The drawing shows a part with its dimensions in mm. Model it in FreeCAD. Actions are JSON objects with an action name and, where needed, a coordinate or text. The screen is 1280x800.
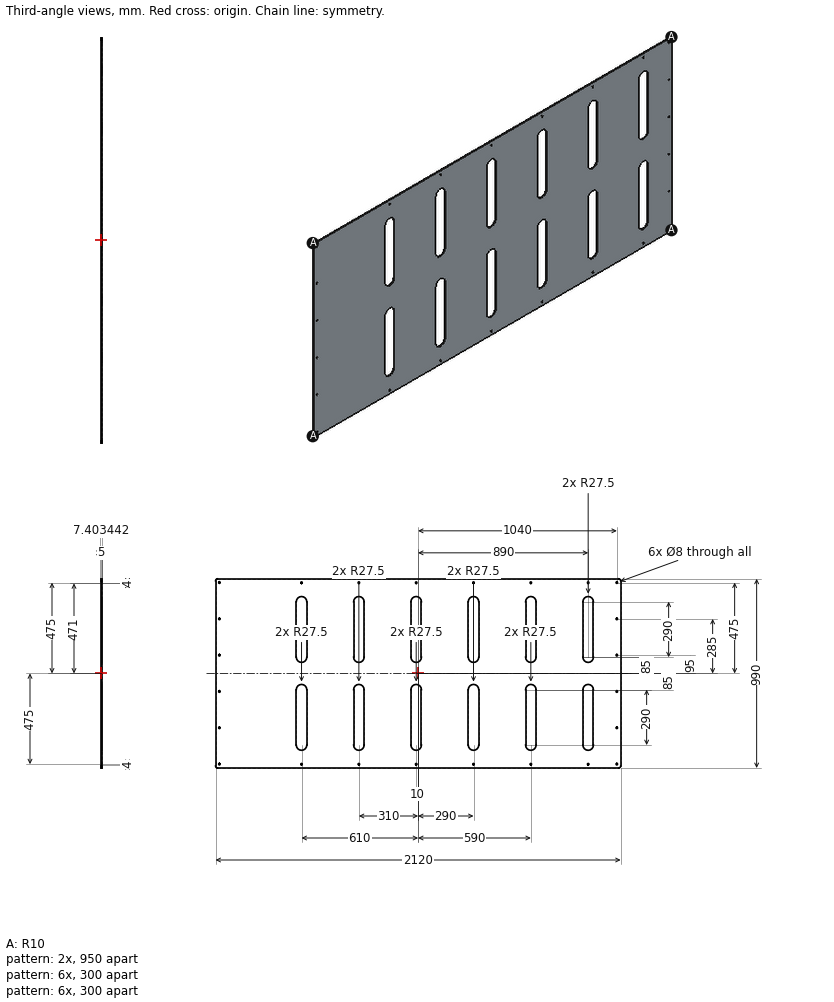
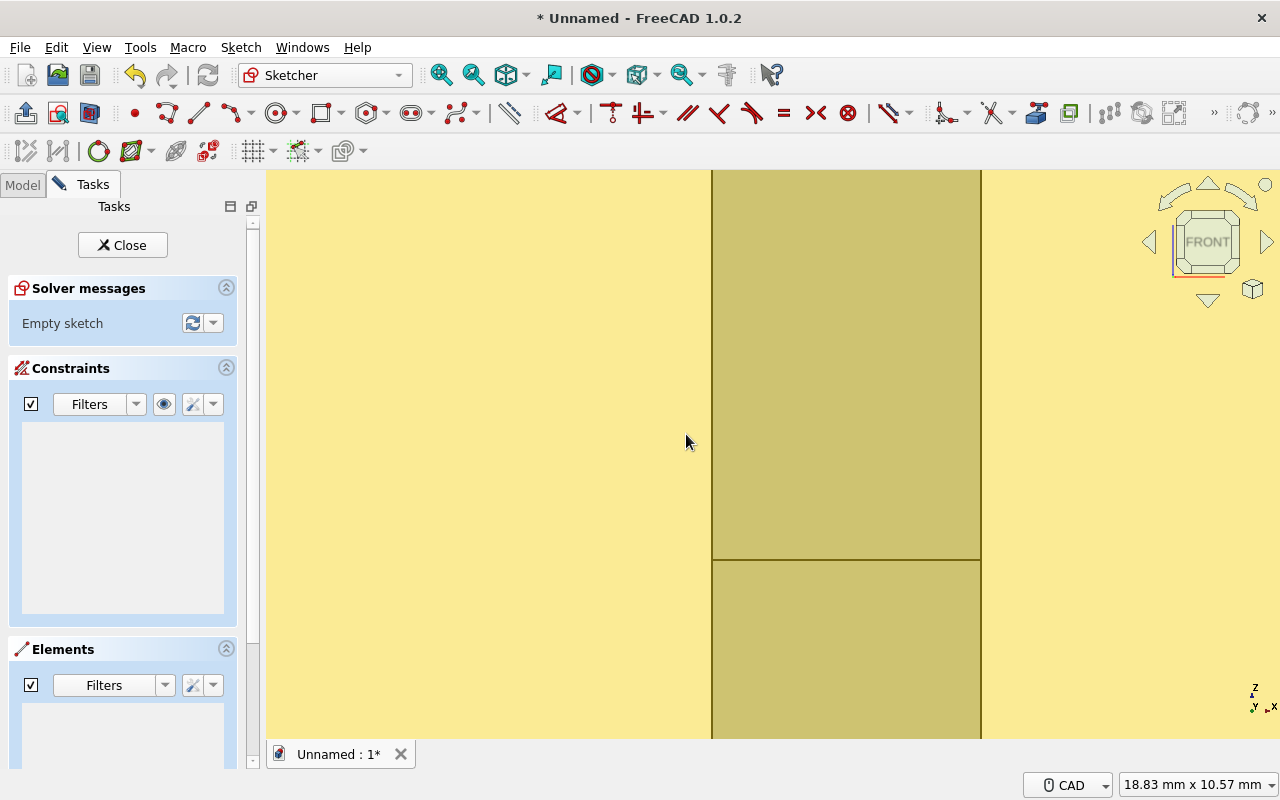
{"action": "left_click", "coordinate": [168, 114]}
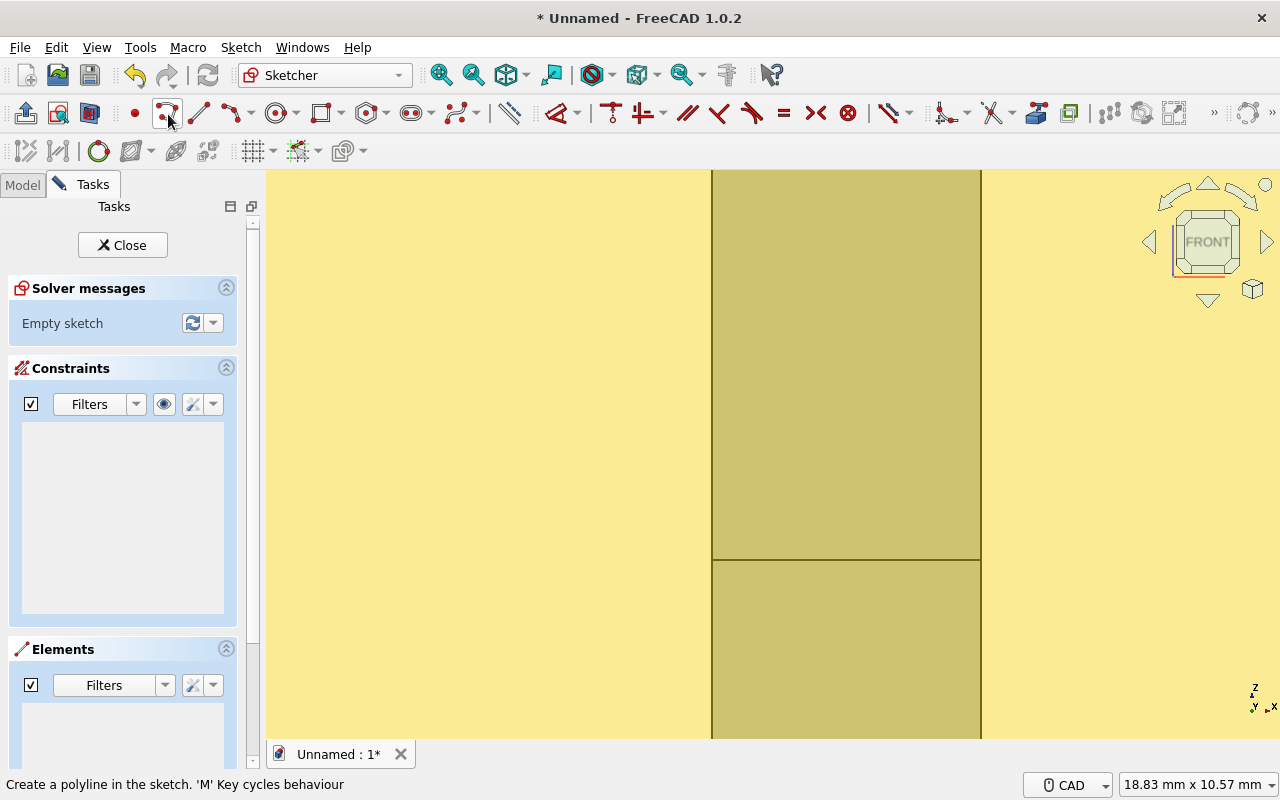
{"action": "left_click", "coordinate": [582, 345]}
{"action": "left_click", "coordinate": [981, 345]}
{"action": "left_click", "coordinate": [981, 560]}
{"action": "left_click", "coordinate": [712, 560]}
{"action": "left_click", "coordinate": [582, 346]}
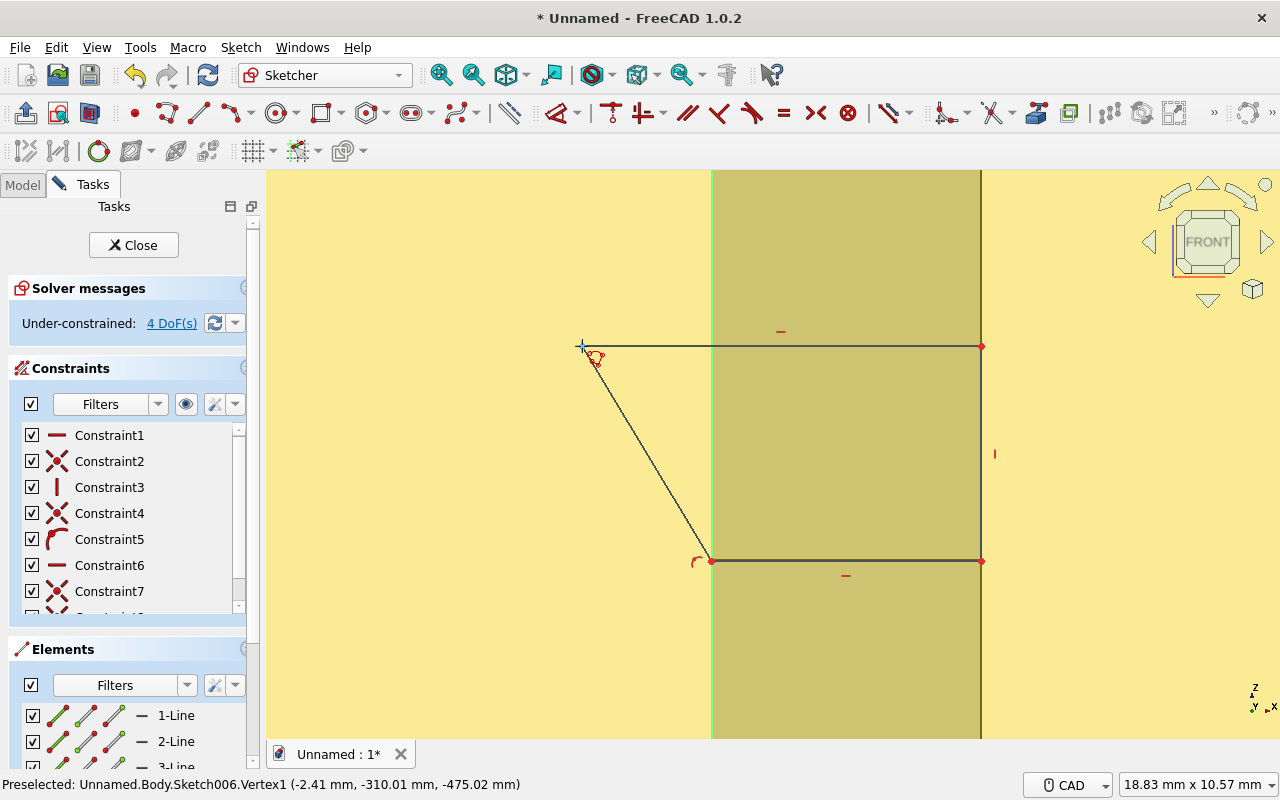
{"action": "left_click", "coordinate": [200, 114]}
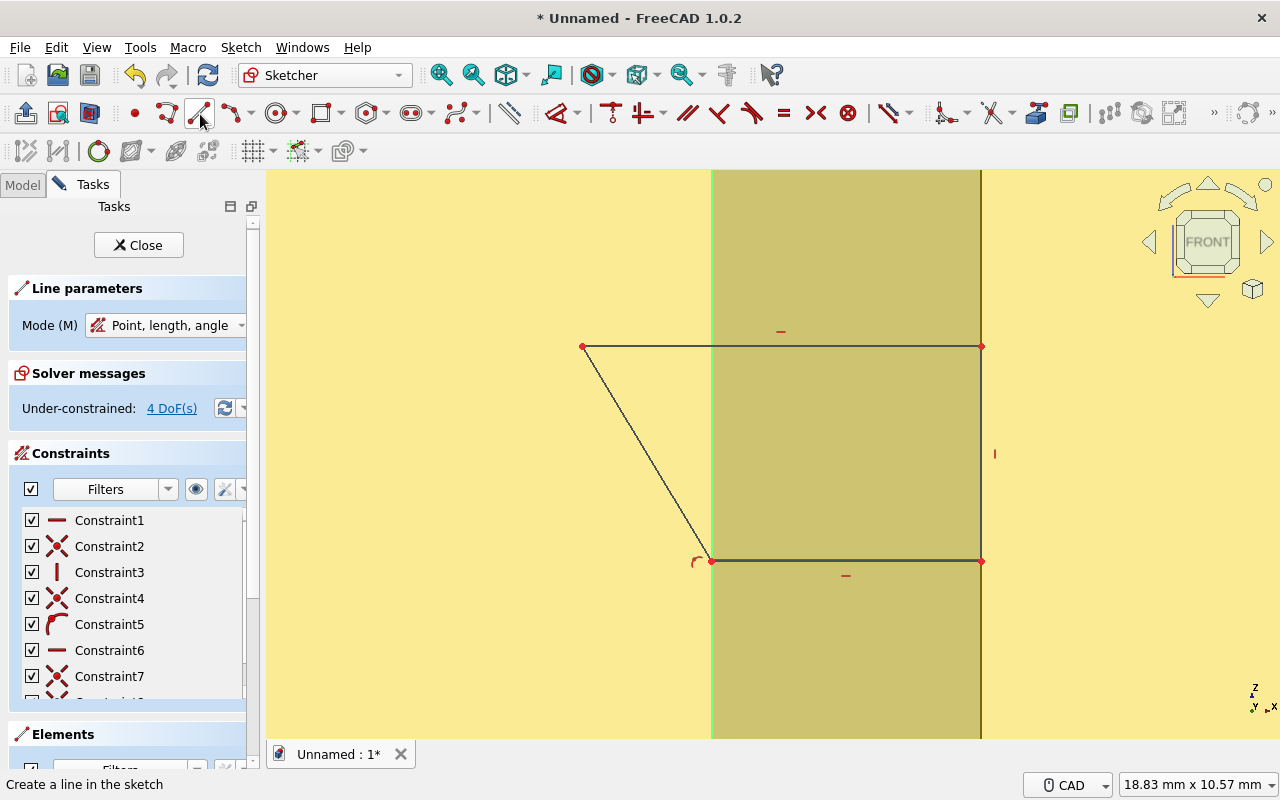
{"action": "left_click", "coordinate": [542, 345]}
{"action": "left_click", "coordinate": [423, 345]}
{"action": "key", "text": "Escape"}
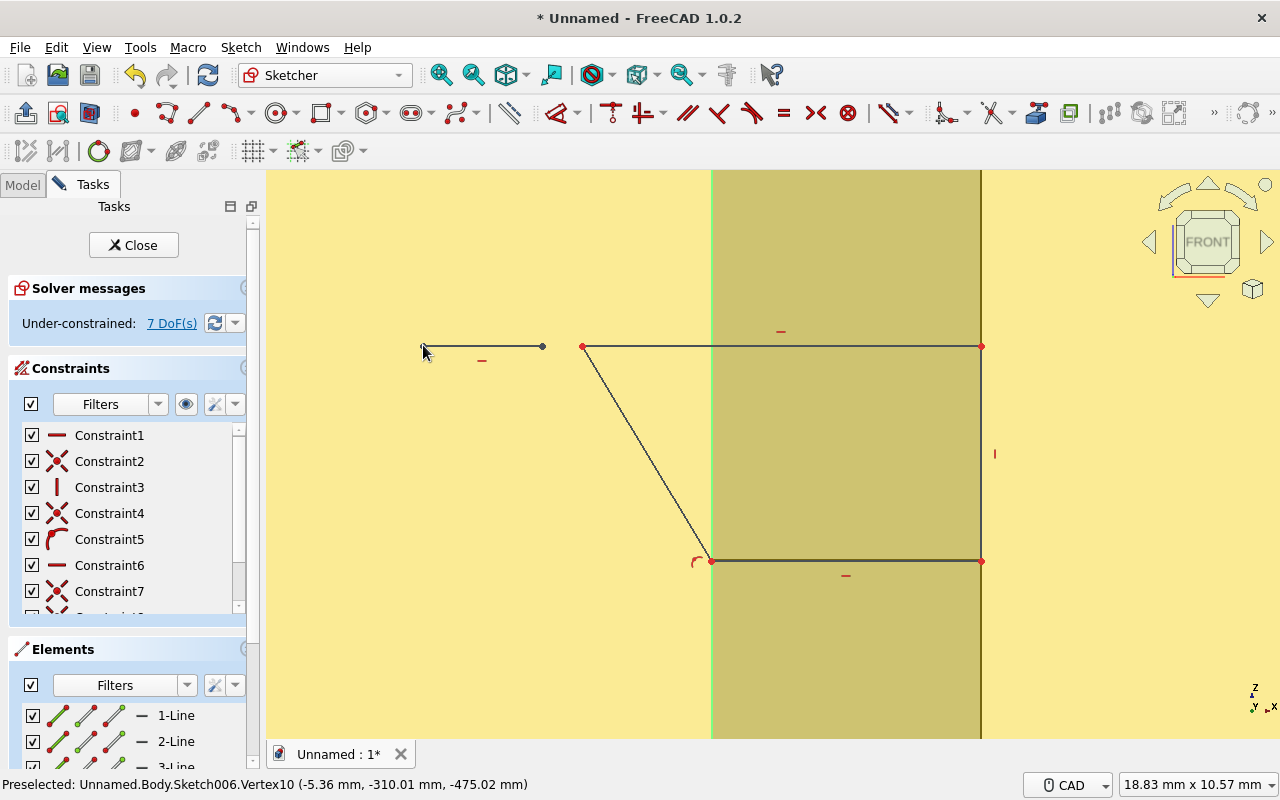
{"action": "left_click", "coordinate": [506, 346]}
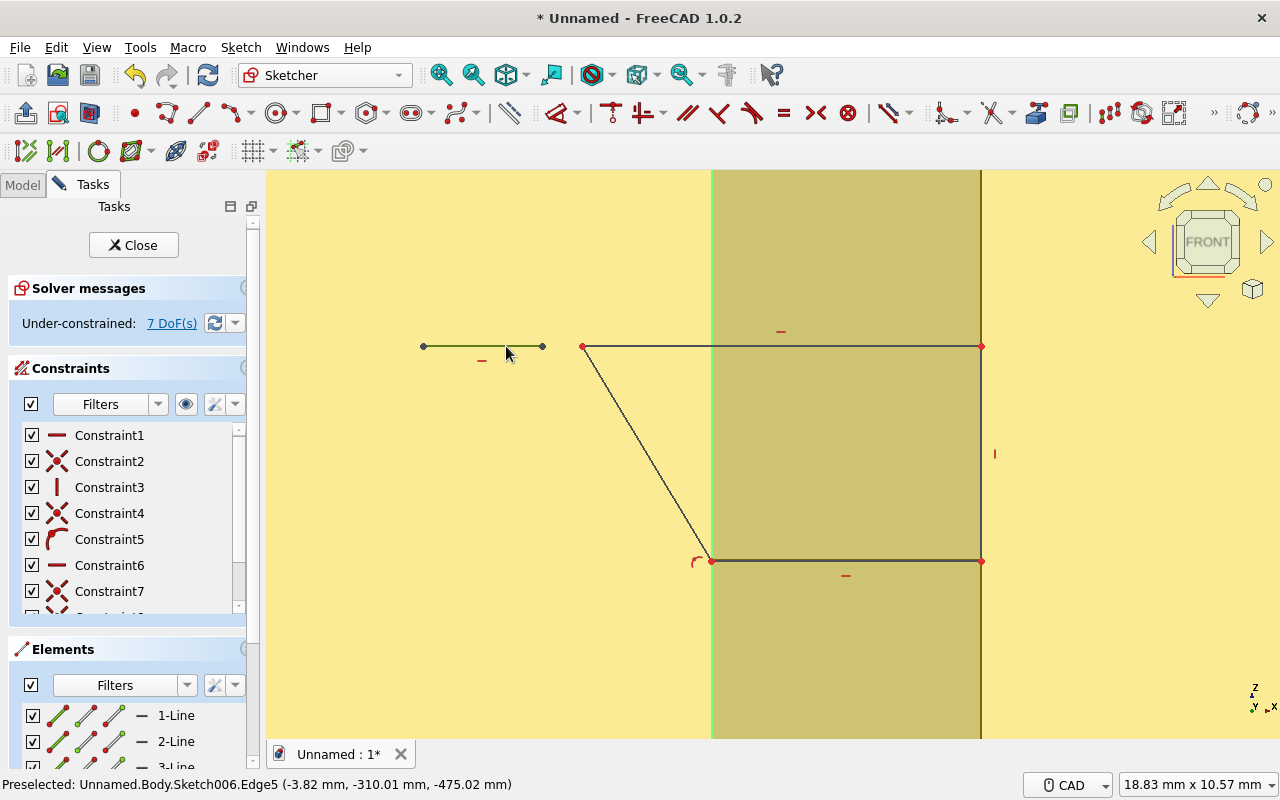
{"action": "left_click", "coordinate": [510, 114]}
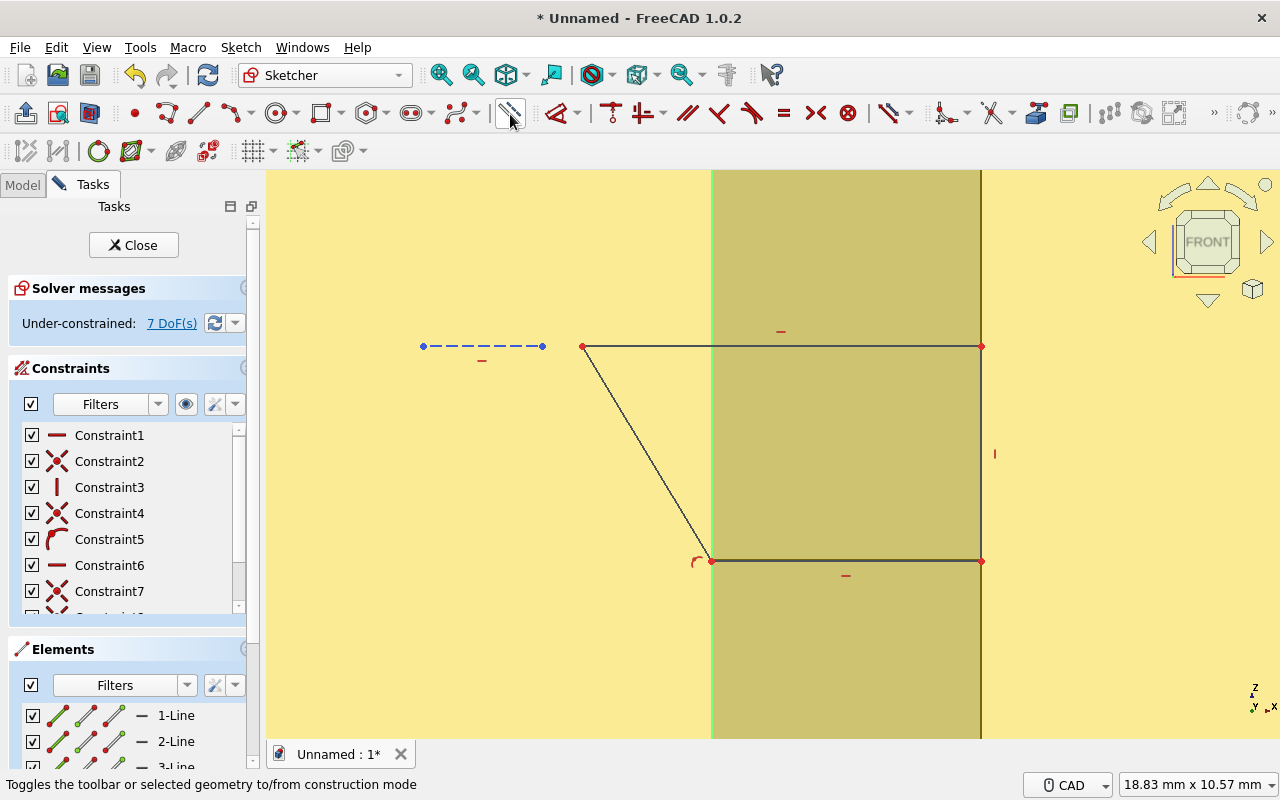
{"action": "left_click", "coordinate": [556, 114]}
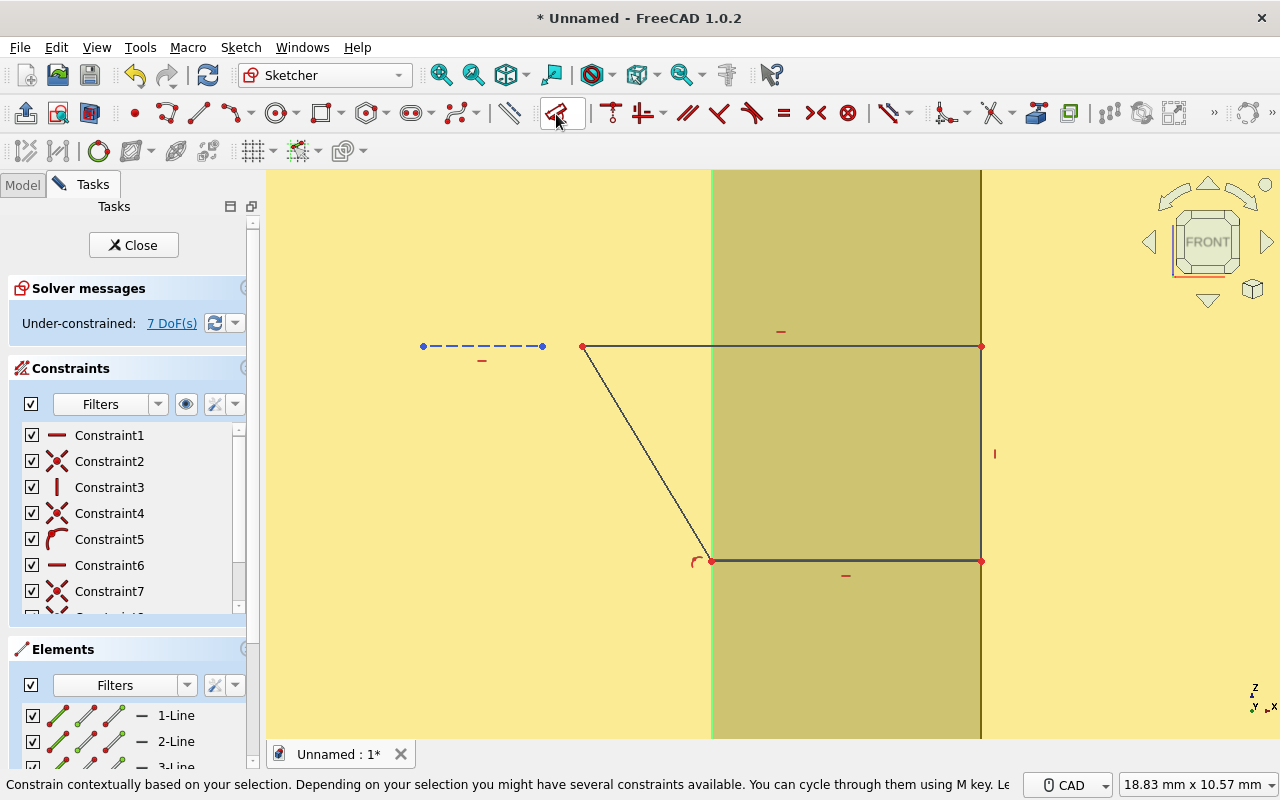
{"action": "left_click", "coordinate": [981, 411]}
{"action": "left_click", "coordinate": [1015, 454]}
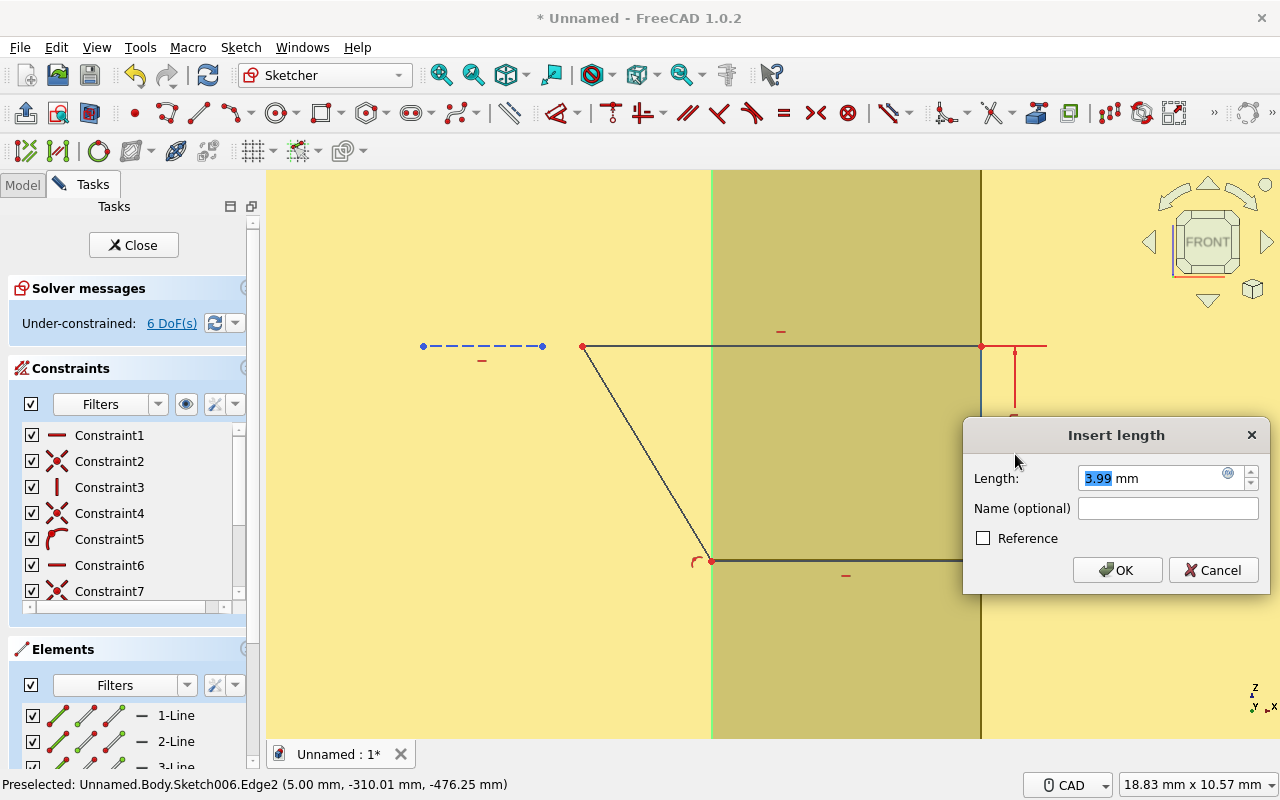
{"action": "type", "text": "4"}
{"action": "key", "text": "Return"}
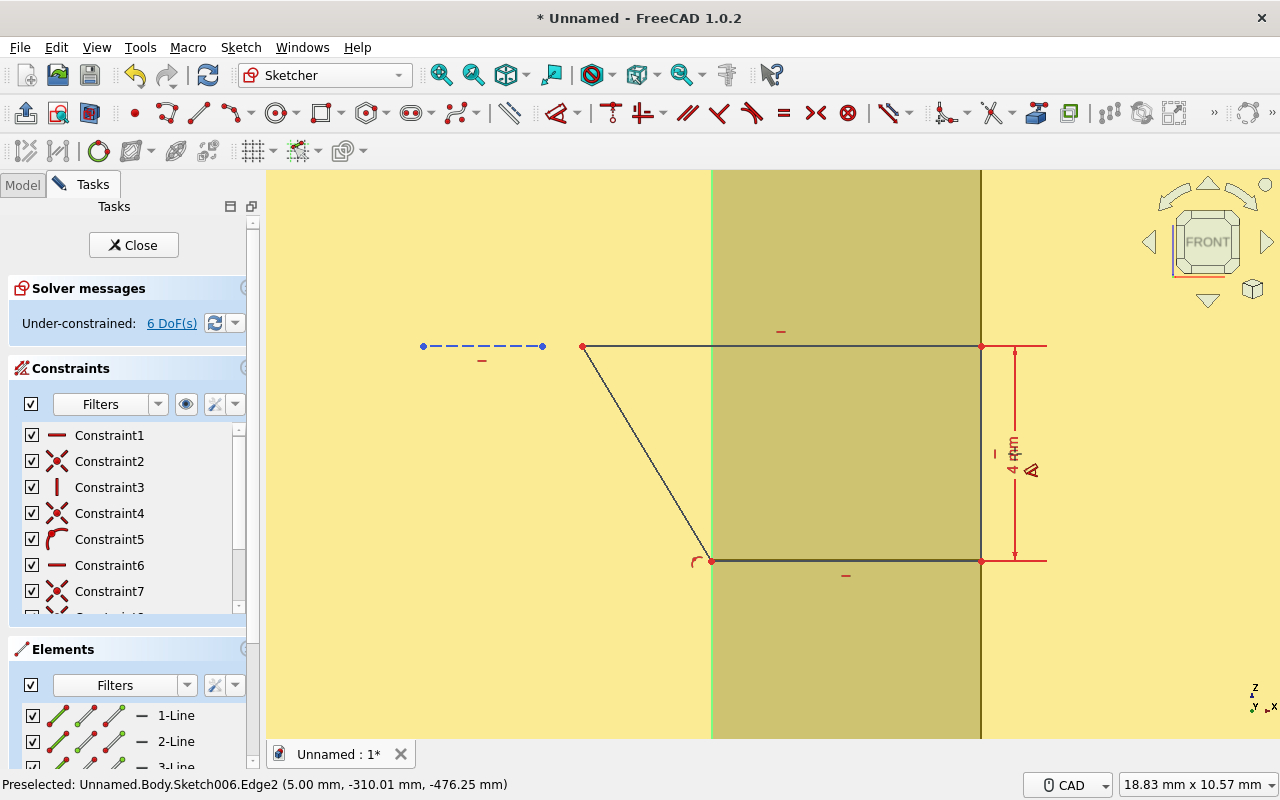
{"action": "left_click", "coordinate": [900, 561]}
{"action": "left_click", "coordinate": [846, 595]}